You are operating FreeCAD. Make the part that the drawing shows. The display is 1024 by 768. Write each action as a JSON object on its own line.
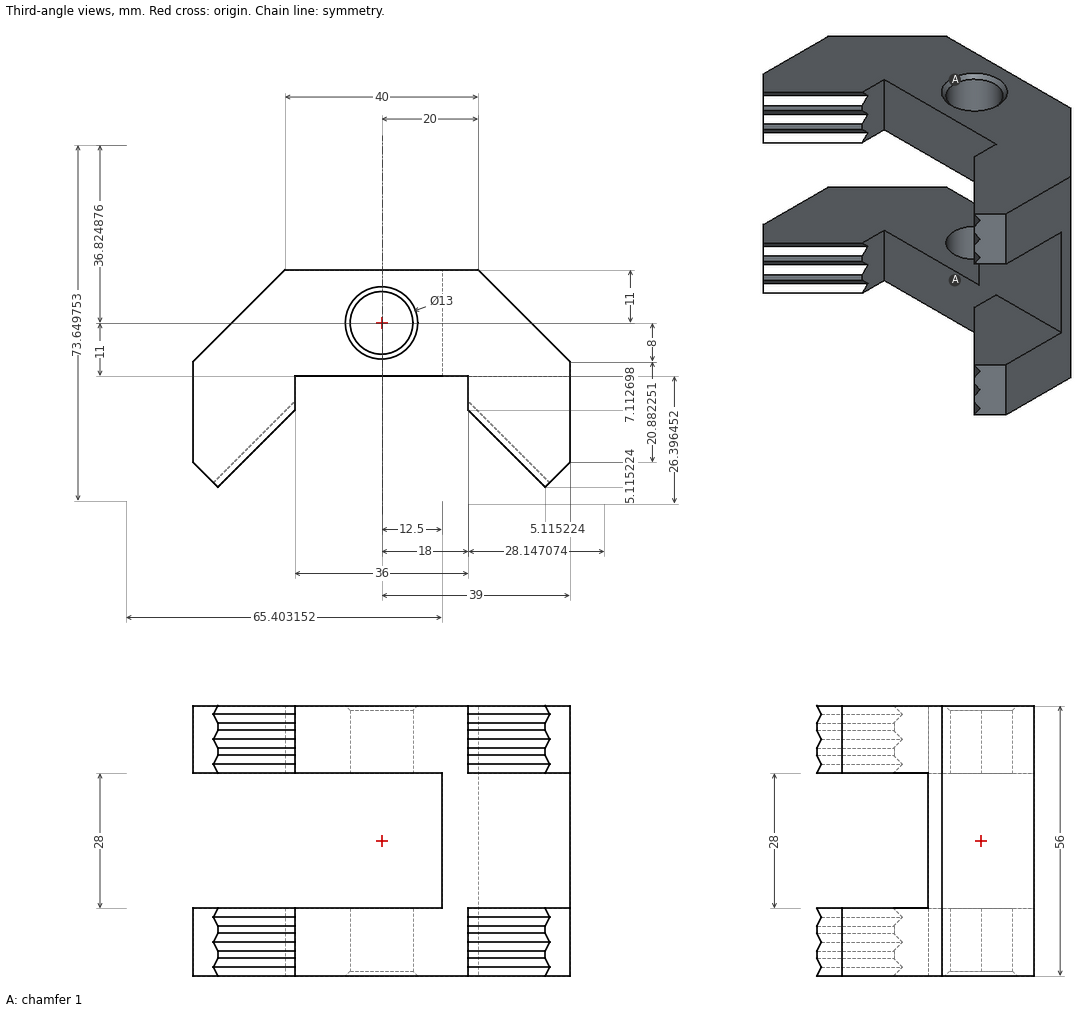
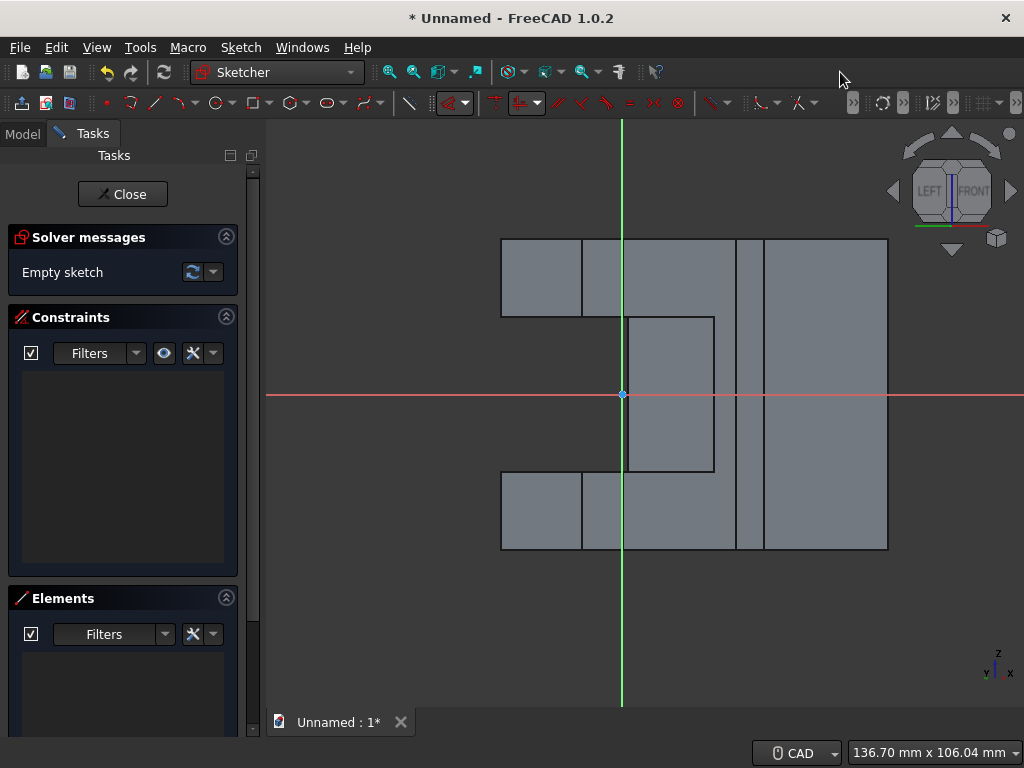
{"action": "scroll", "coordinate": [654, 521], "scroll_direction": "up", "scroll_amount": 4}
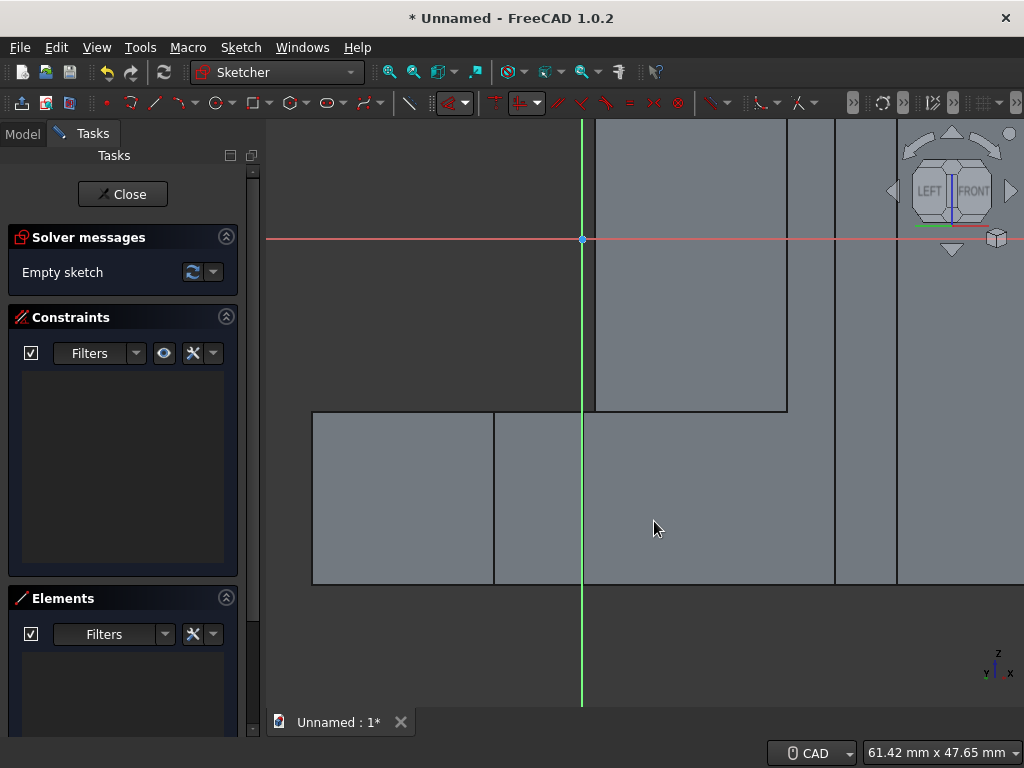
{"action": "left_click", "coordinate": [132, 104]}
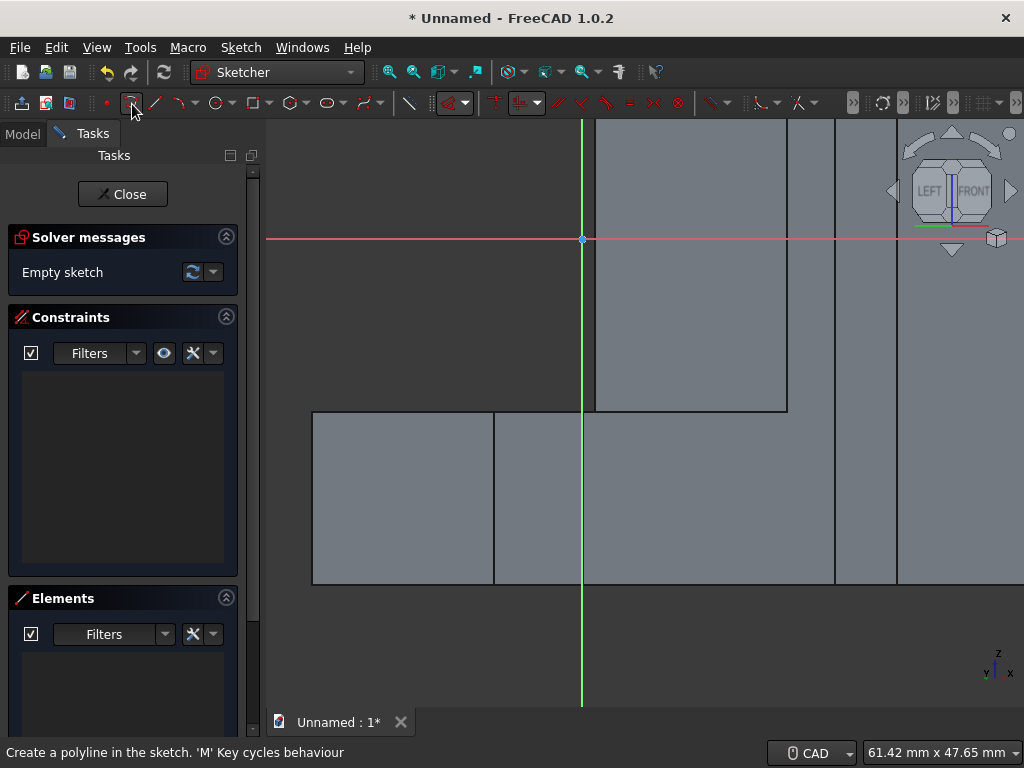
{"action": "scroll", "coordinate": [583, 476], "scroll_direction": "up", "scroll_amount": 14}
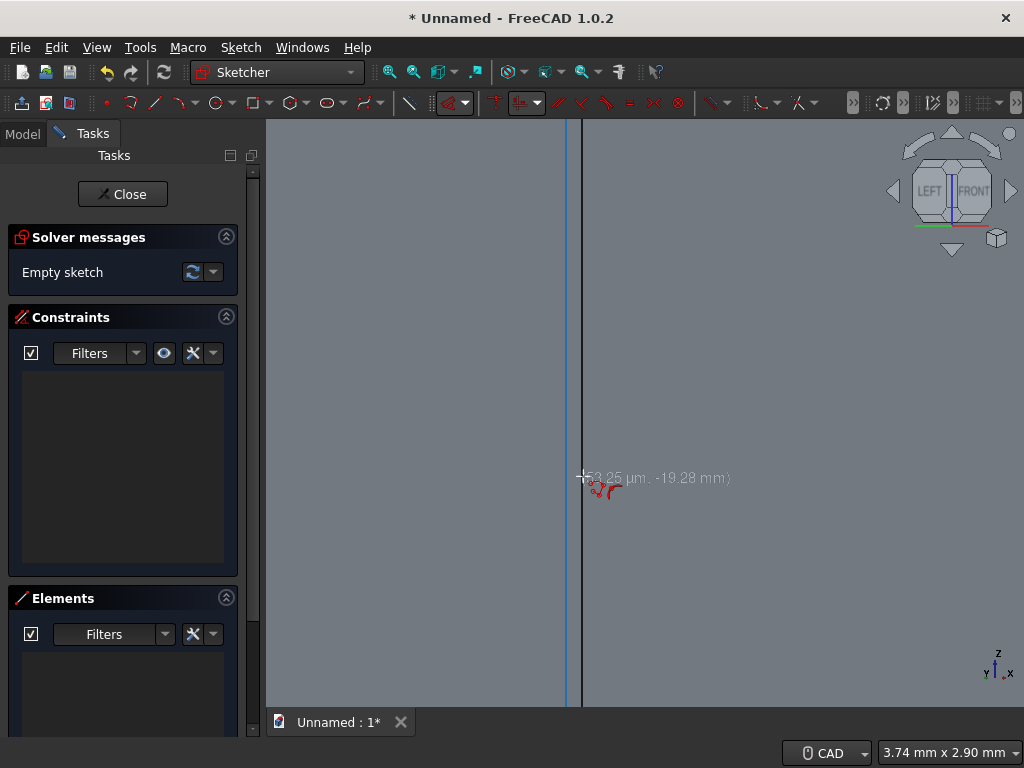
{"action": "left_click", "coordinate": [582, 459]}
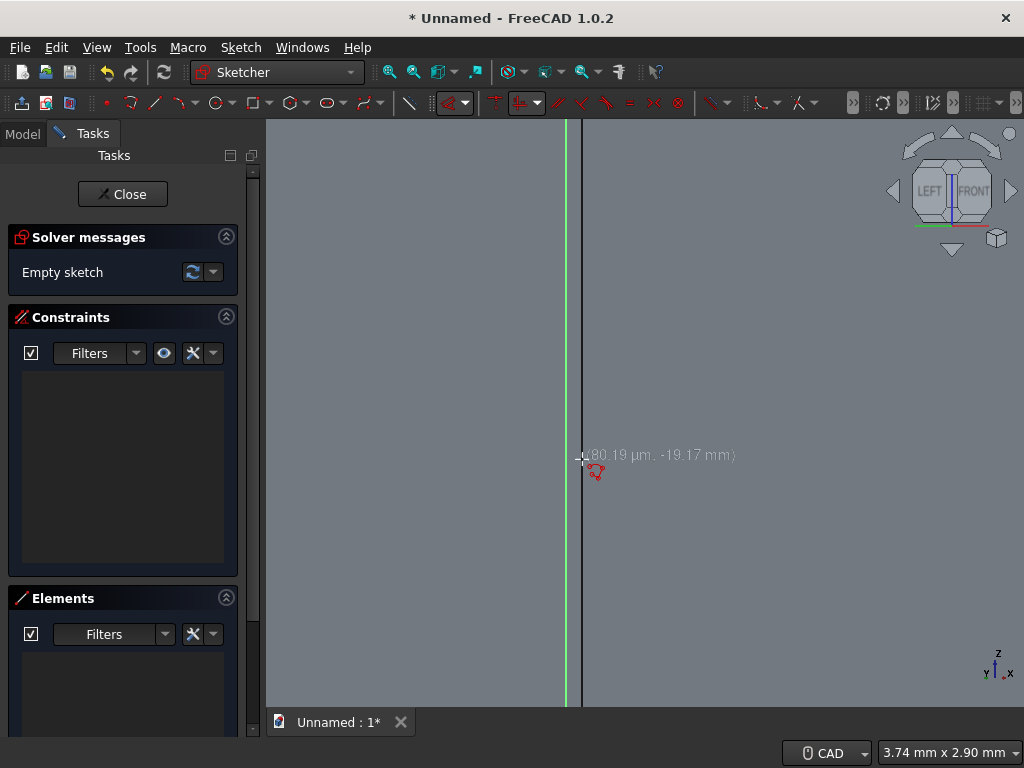
{"action": "scroll", "coordinate": [585, 478], "scroll_direction": "down", "scroll_amount": 14}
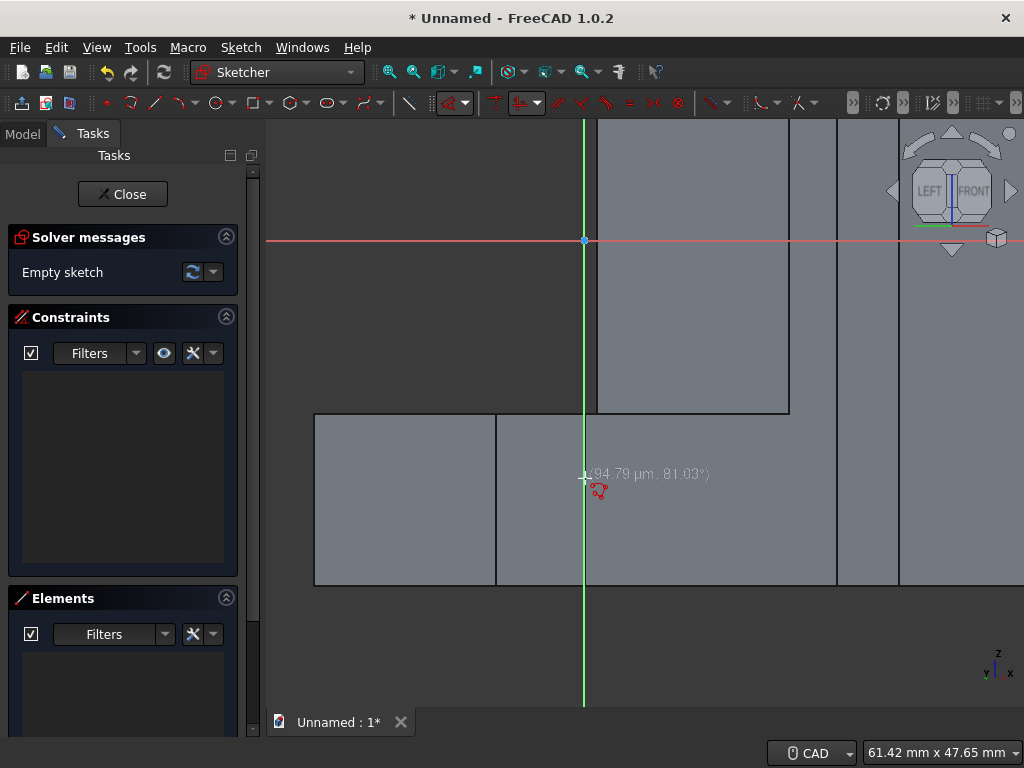
{"action": "left_click", "coordinate": [569, 500]}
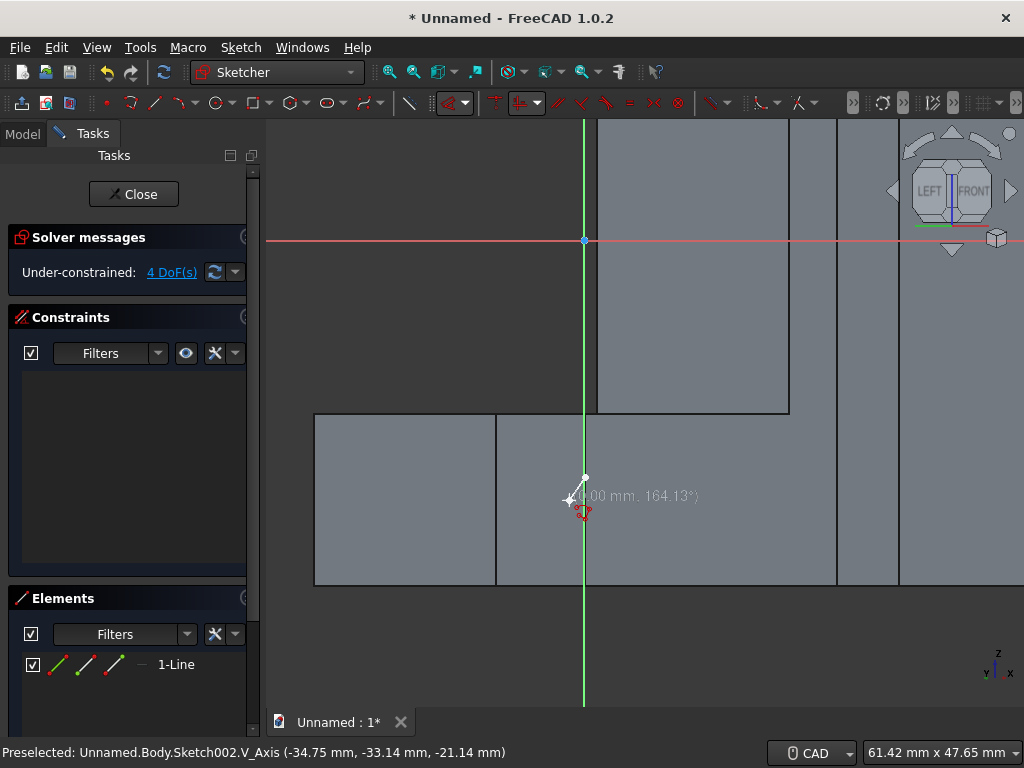
{"action": "scroll", "coordinate": [585, 523], "scroll_direction": "up", "scroll_amount": 14}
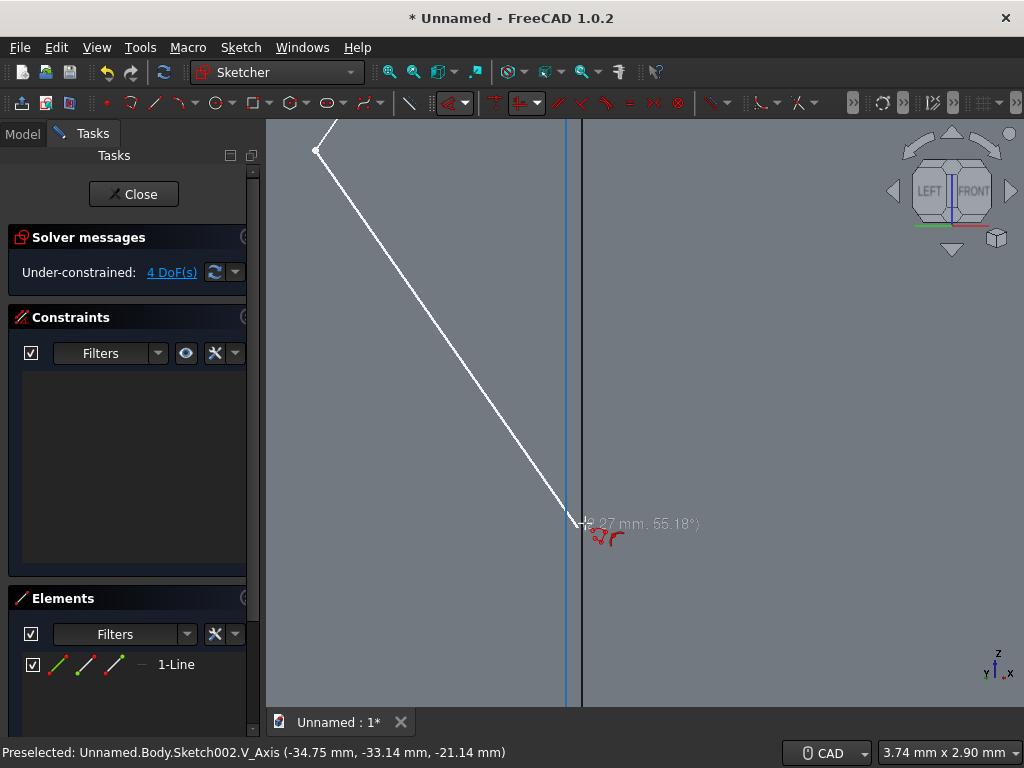
{"action": "left_click", "coordinate": [582, 507]}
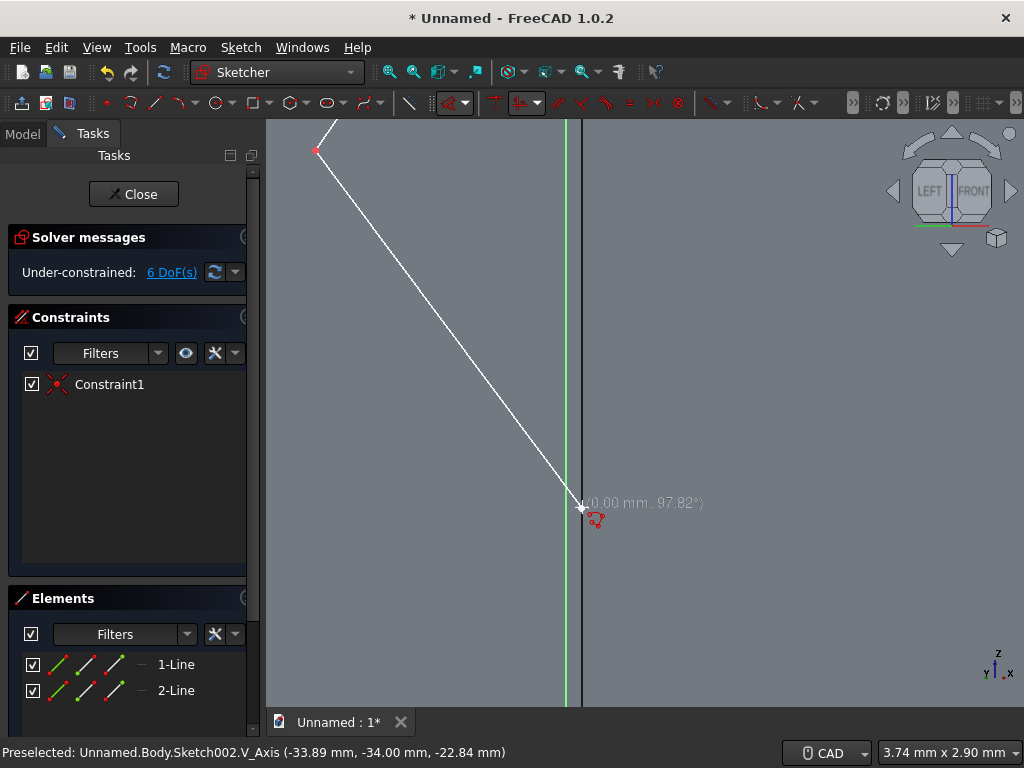
{"action": "scroll", "coordinate": [585, 523], "scroll_direction": "down", "scroll_amount": 14}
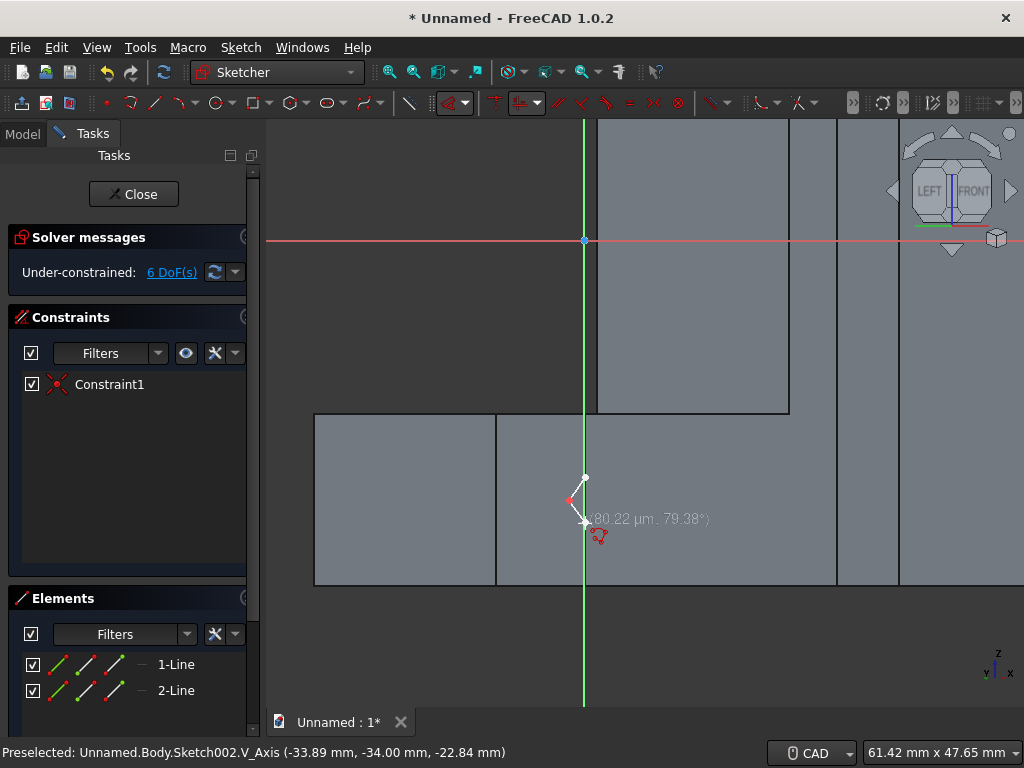
{"action": "scroll", "coordinate": [585, 477], "scroll_direction": "up", "scroll_amount": 14}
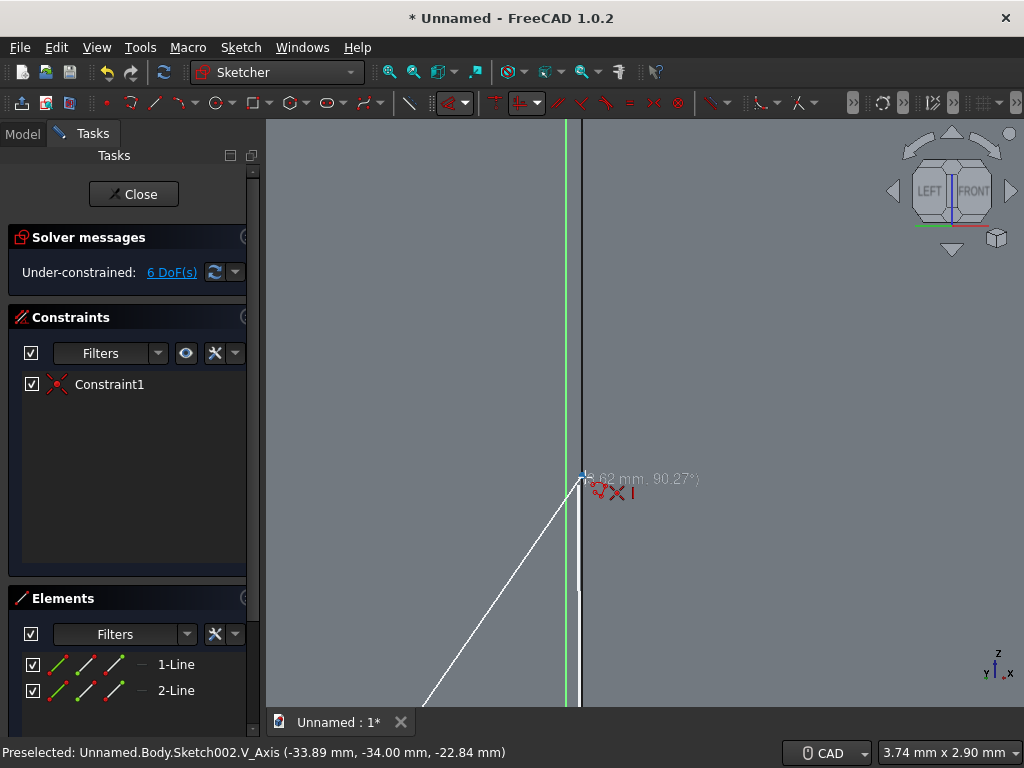
{"action": "left_click", "coordinate": [582, 475]}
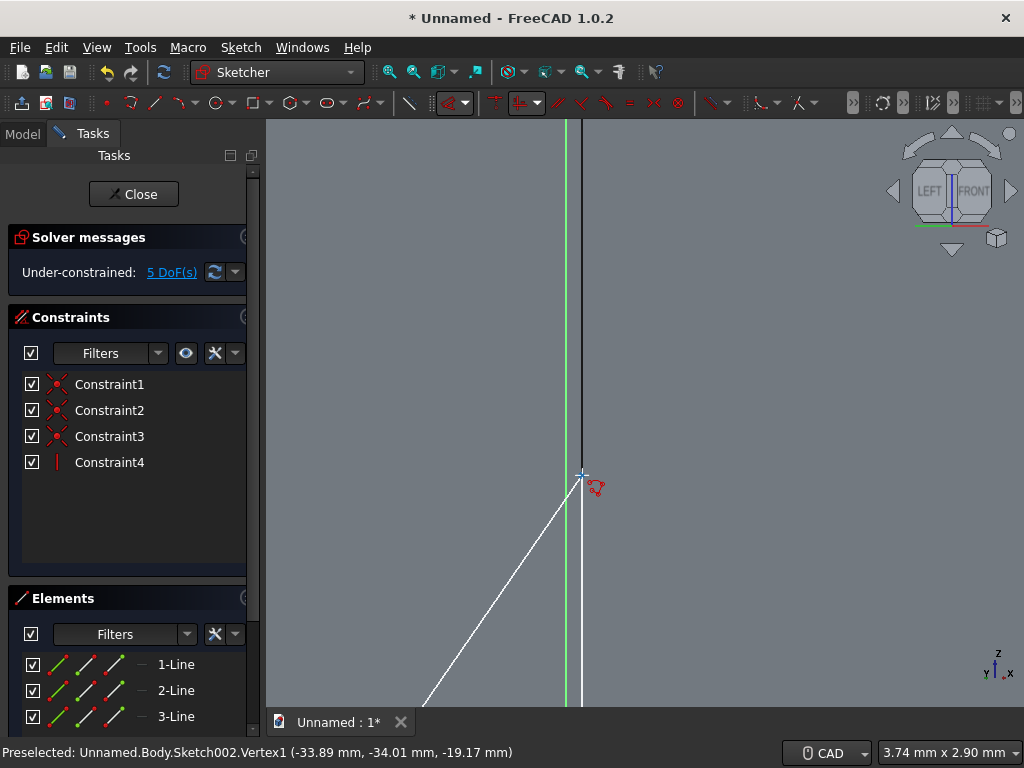
{"action": "scroll", "coordinate": [585, 477], "scroll_direction": "down", "scroll_amount": 14}